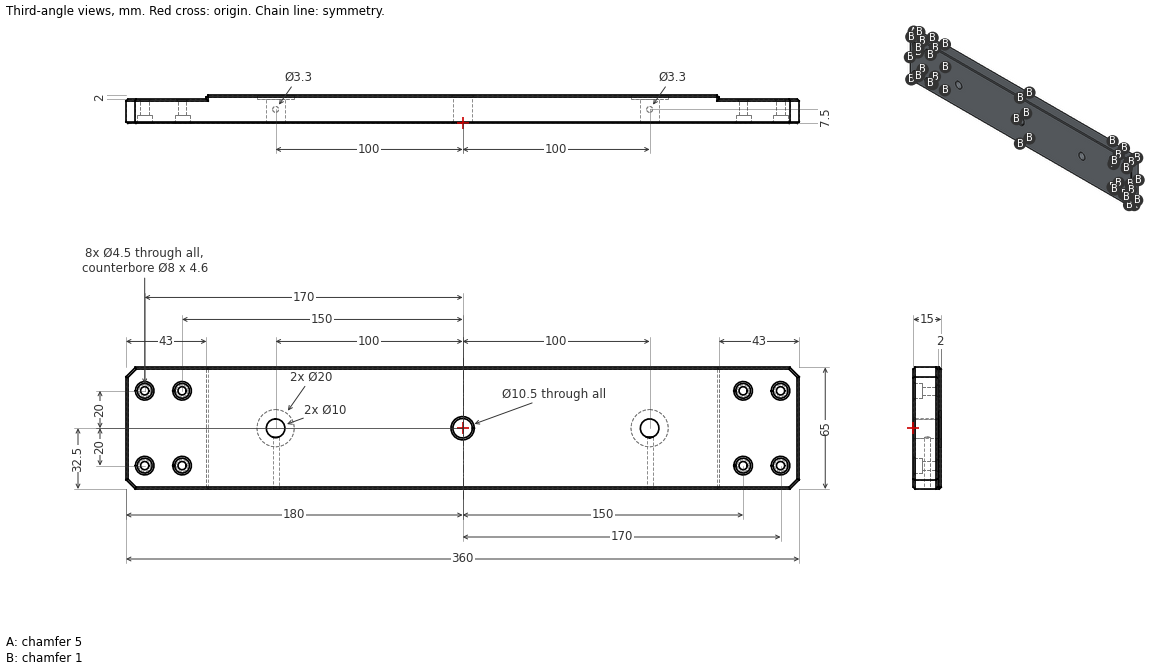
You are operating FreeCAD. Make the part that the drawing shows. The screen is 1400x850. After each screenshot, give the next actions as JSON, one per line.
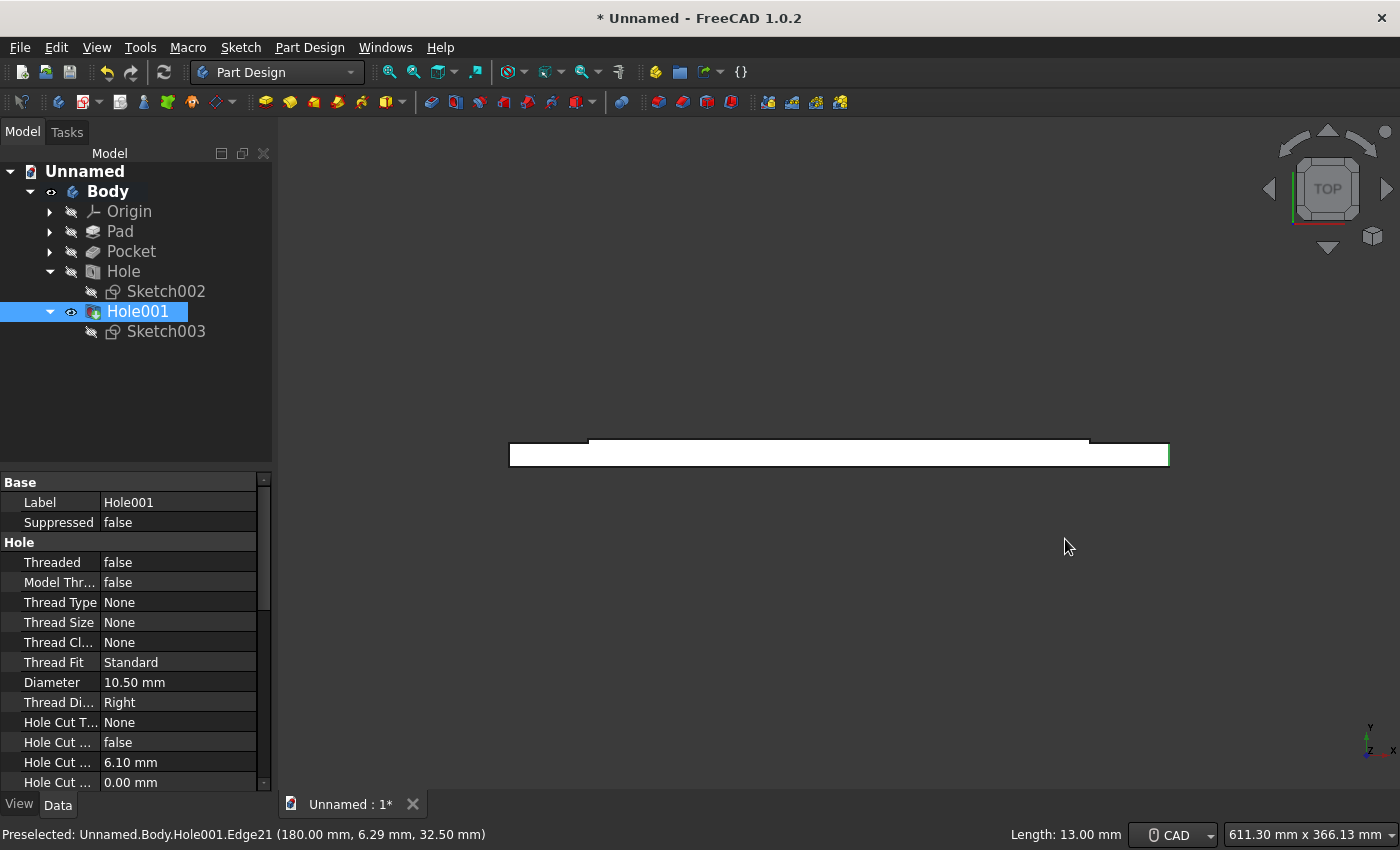
{"action": "left_click", "coordinate": [509, 454], "text": "ctrl"}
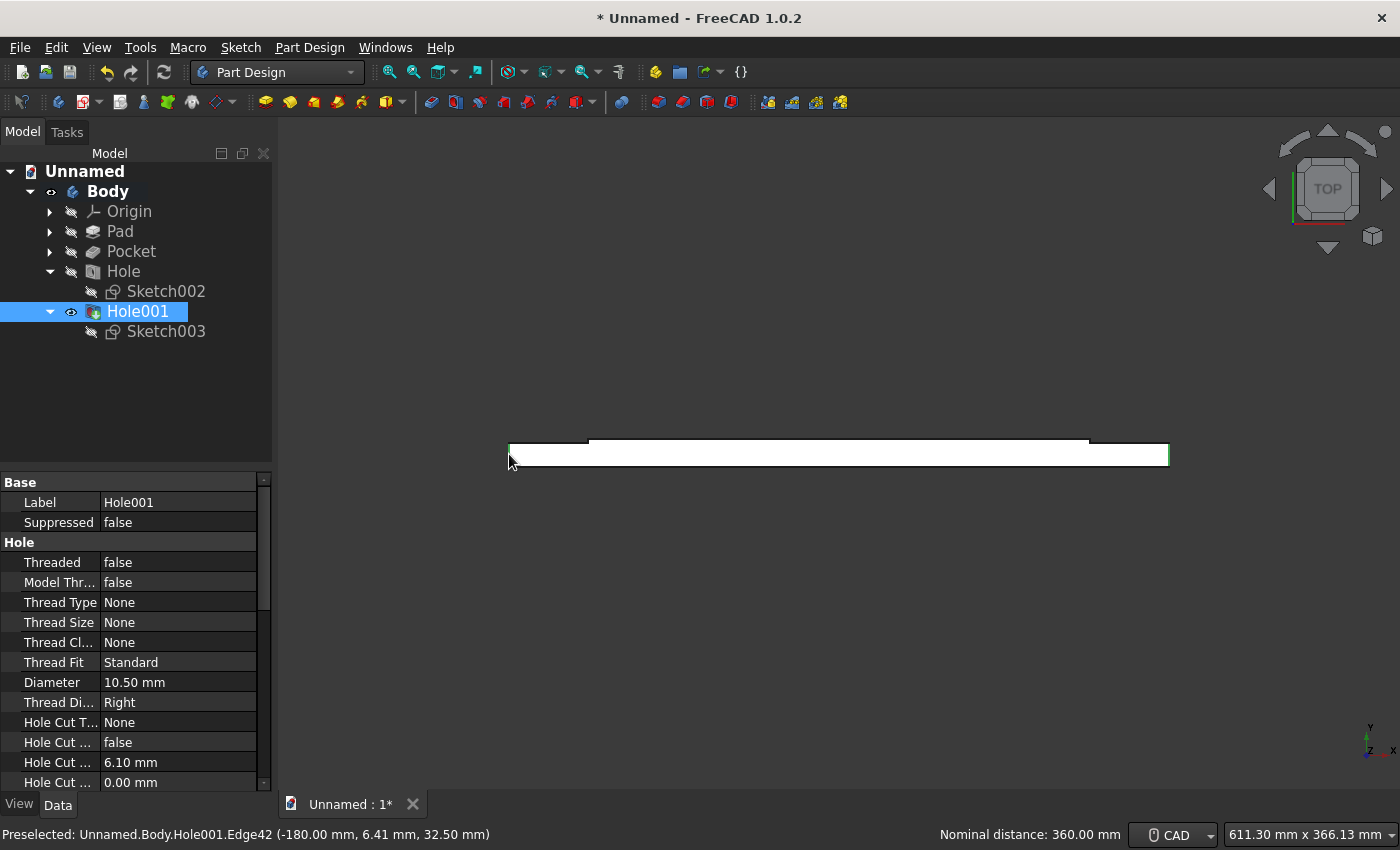
{"action": "key", "text": "1"}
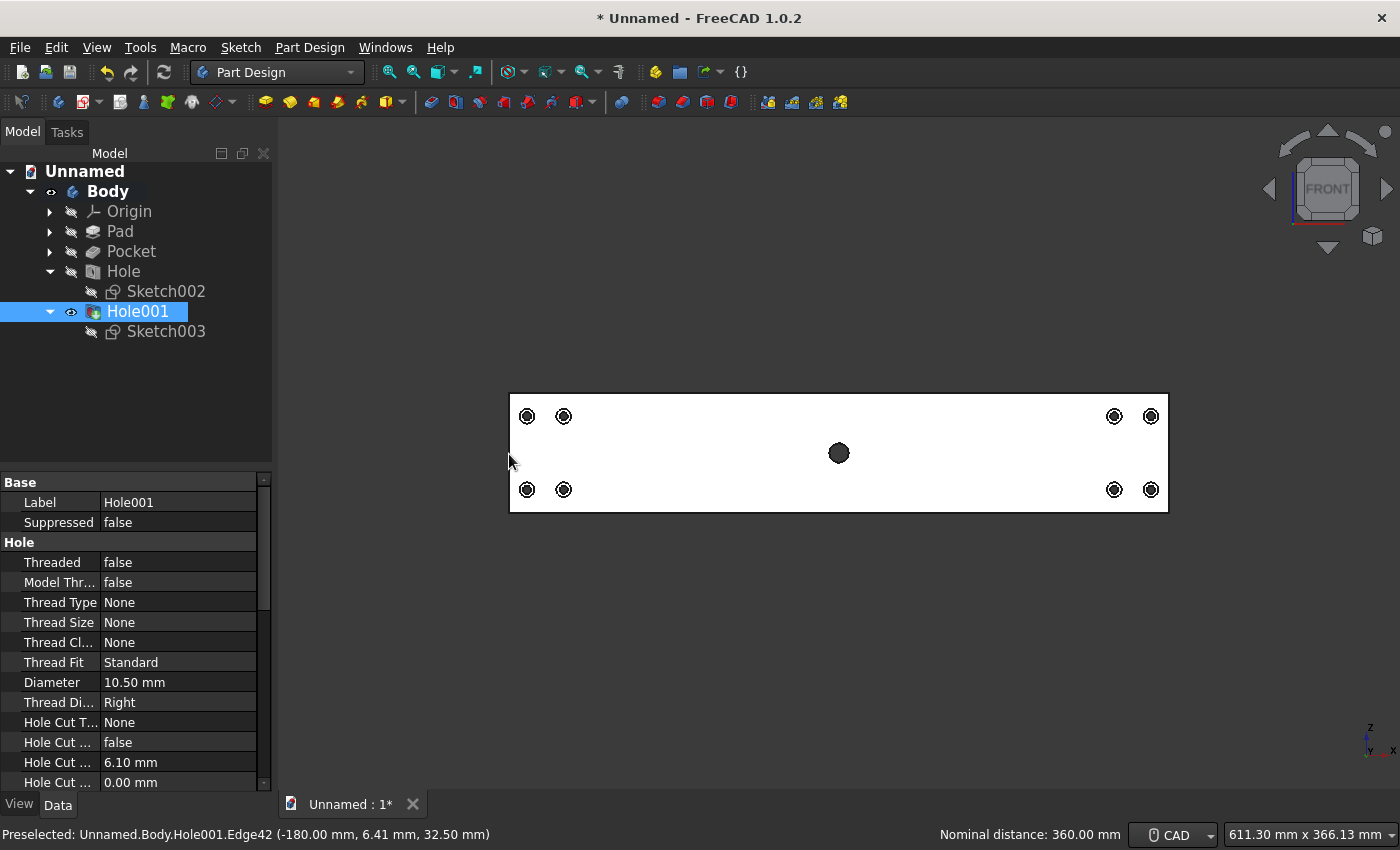
{"action": "key", "text": "3"}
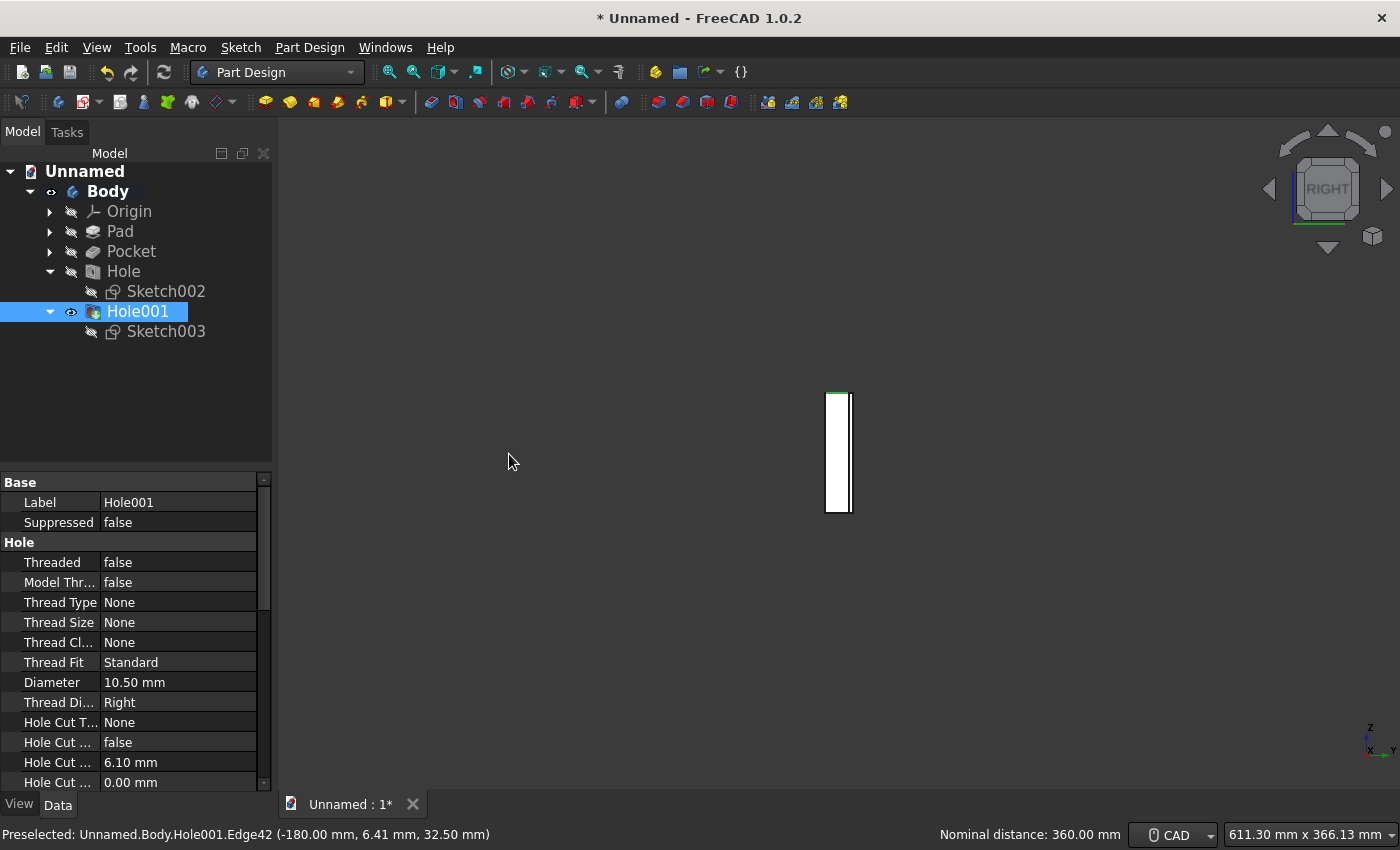
{"action": "key", "text": "v f"}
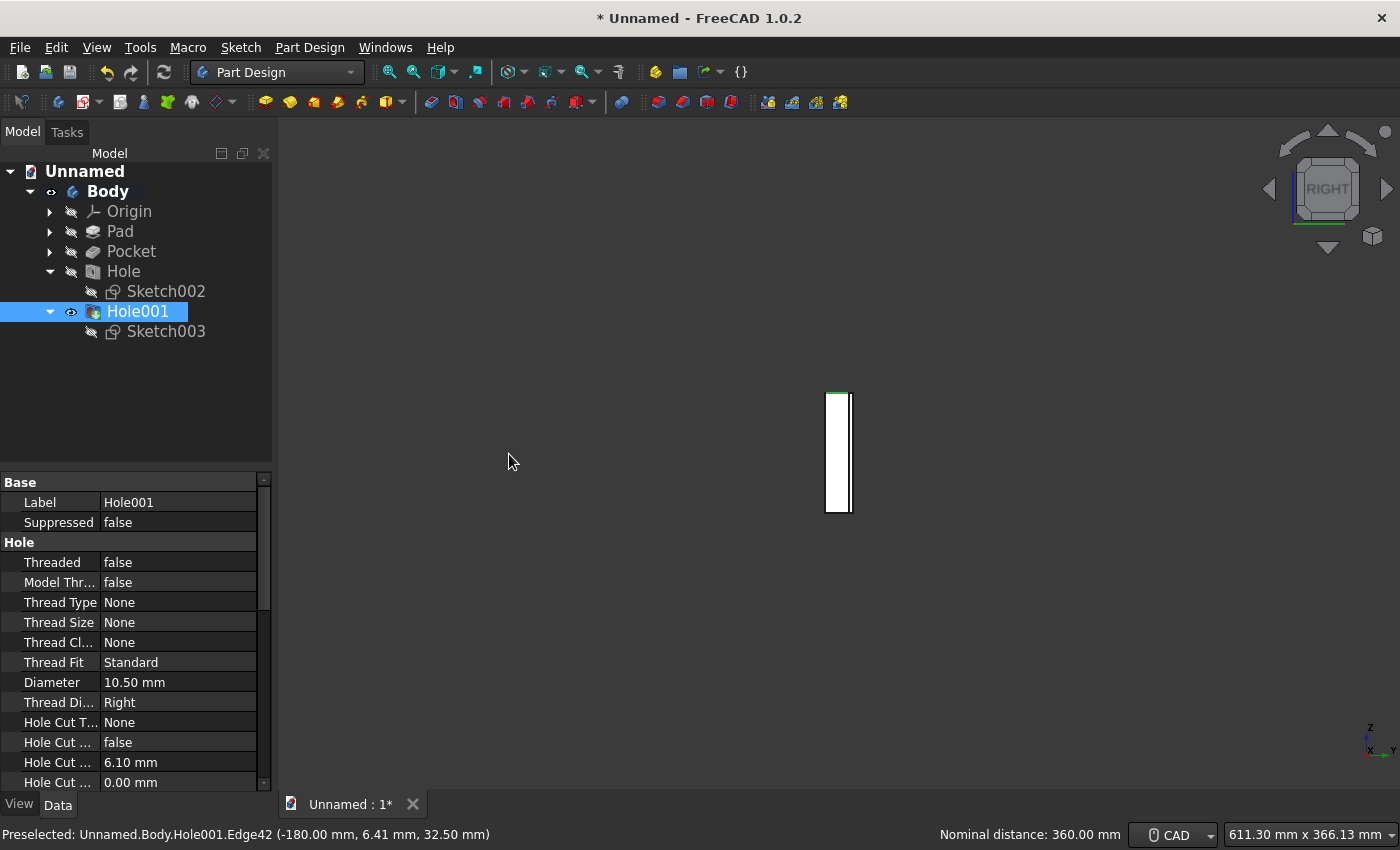
{"action": "left_click", "coordinate": [837, 512], "text": "ctrl"}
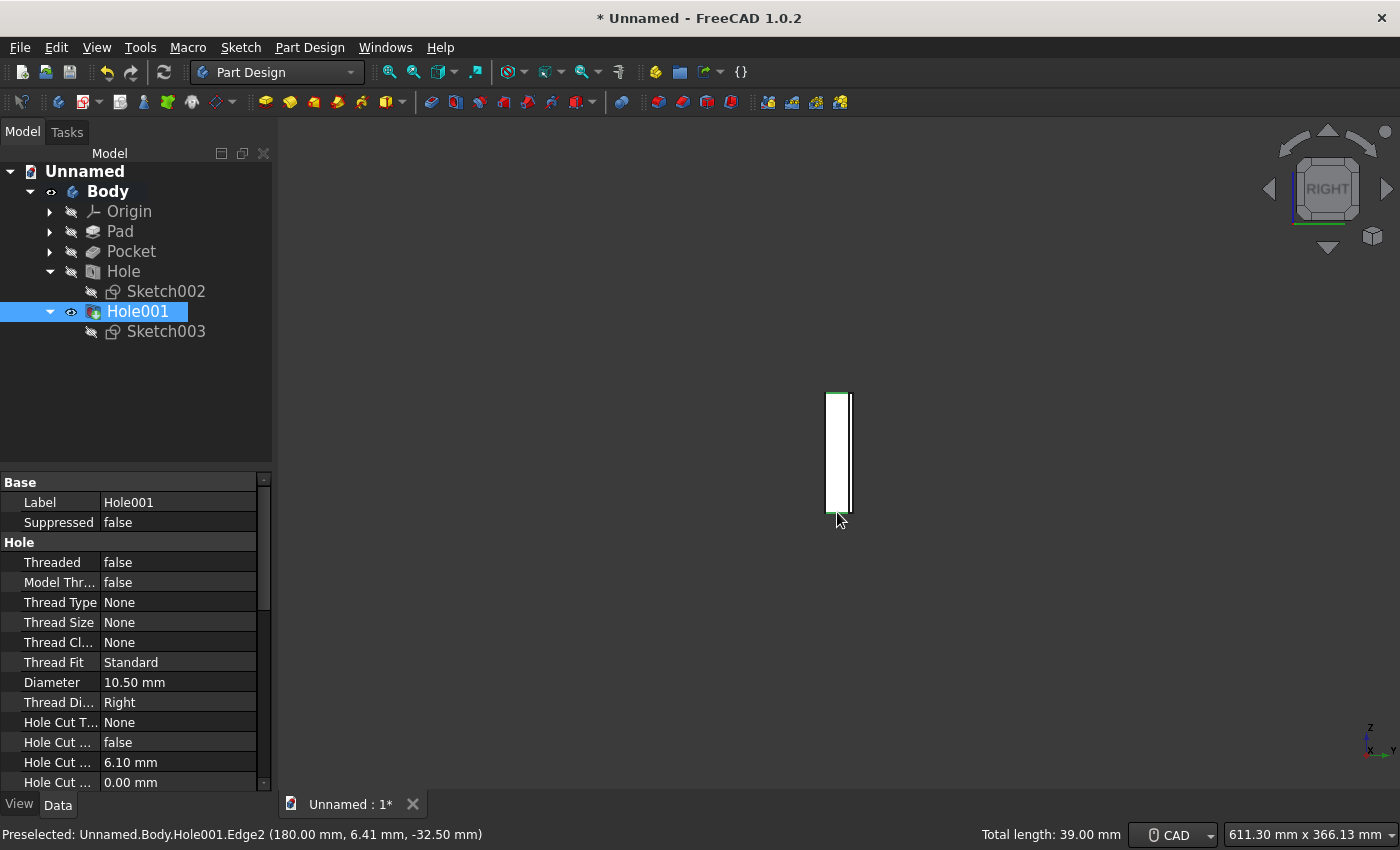
{"action": "key", "text": "5"}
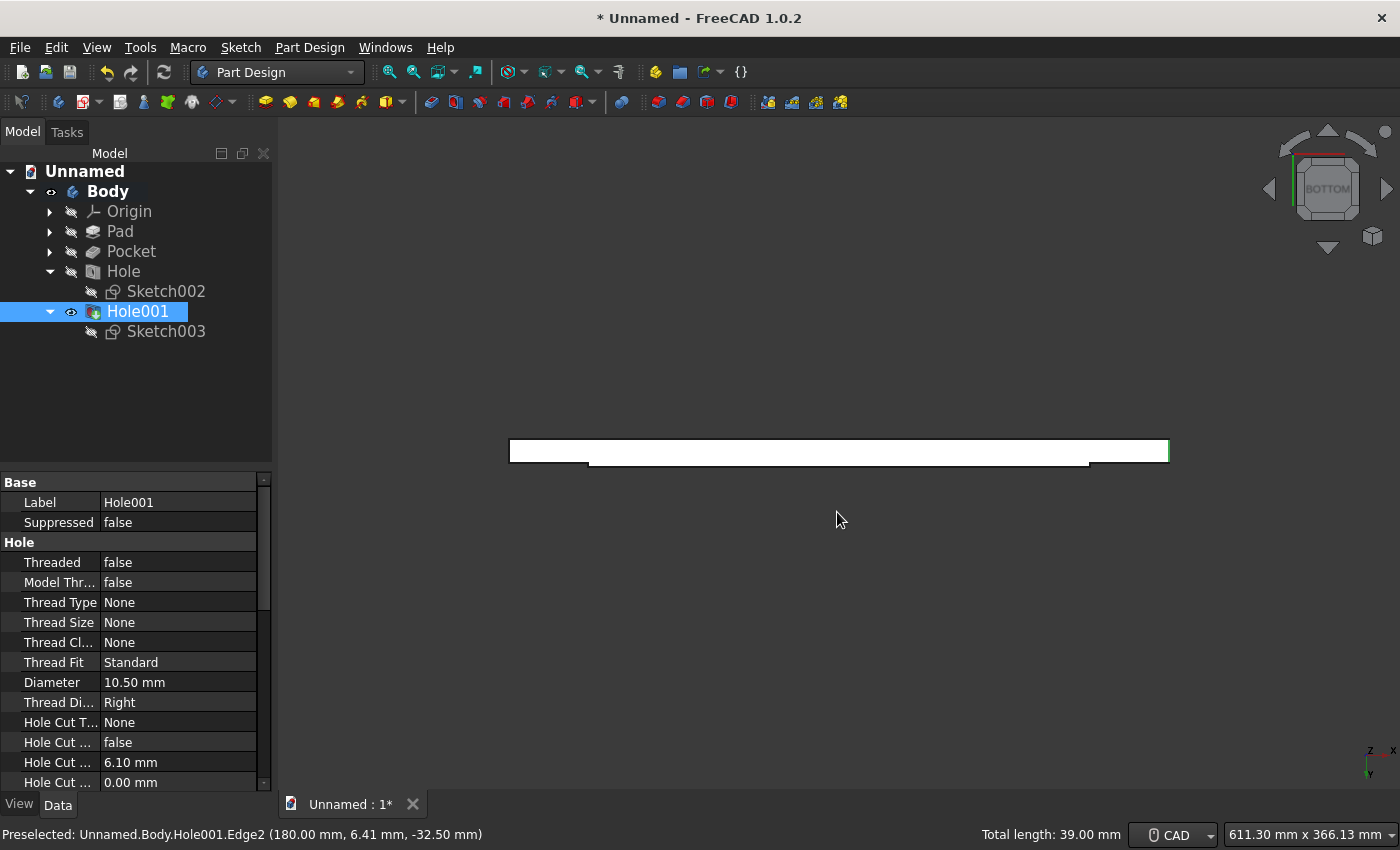
{"action": "left_click", "coordinate": [509, 450], "text": "ctrl"}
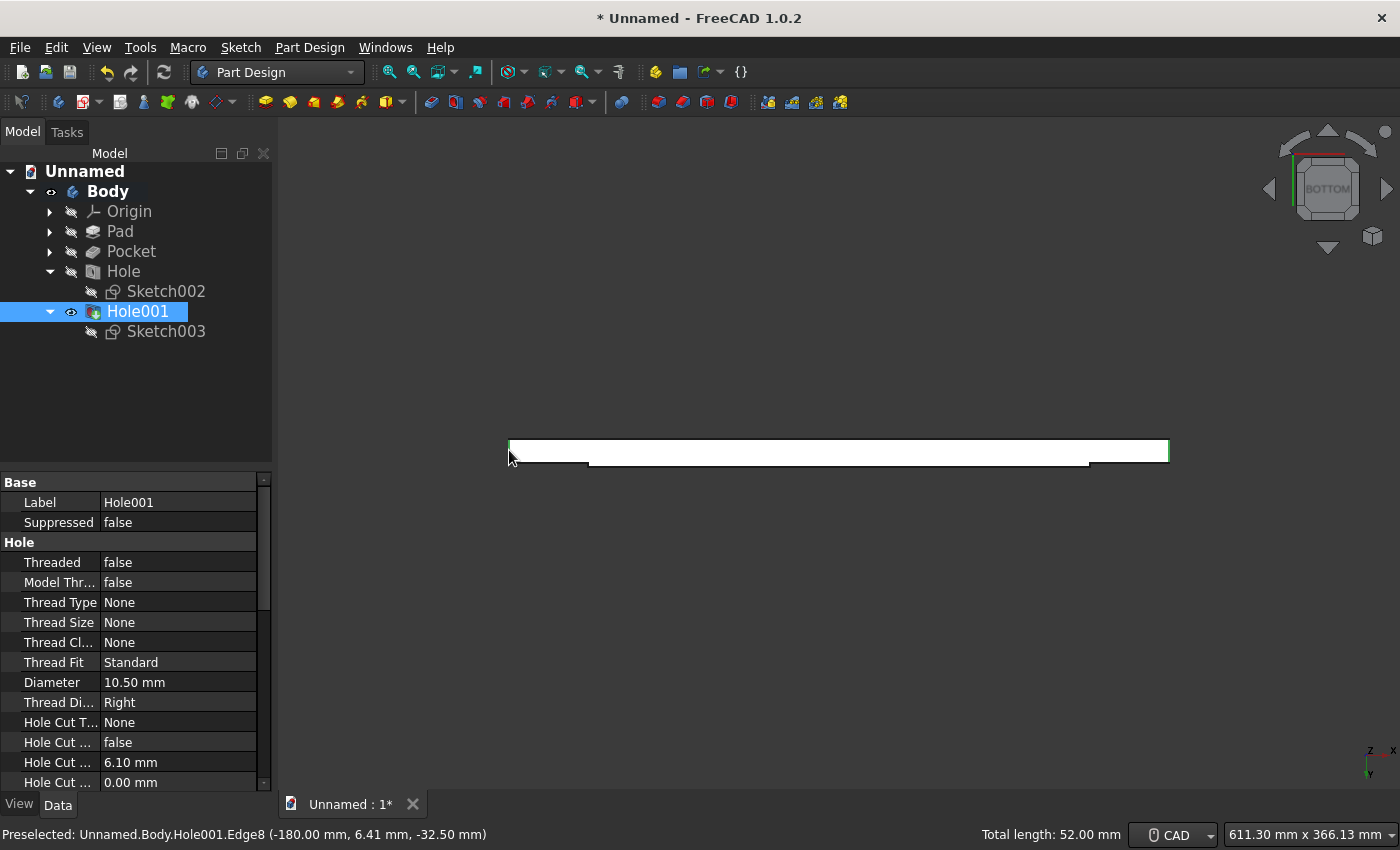
{"action": "left_click", "coordinate": [684, 102]}